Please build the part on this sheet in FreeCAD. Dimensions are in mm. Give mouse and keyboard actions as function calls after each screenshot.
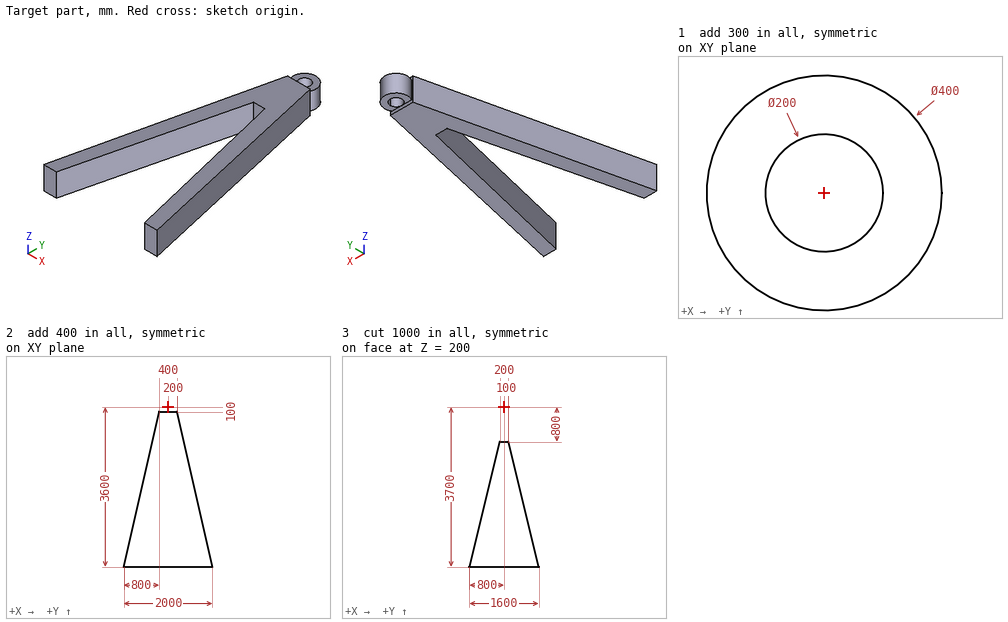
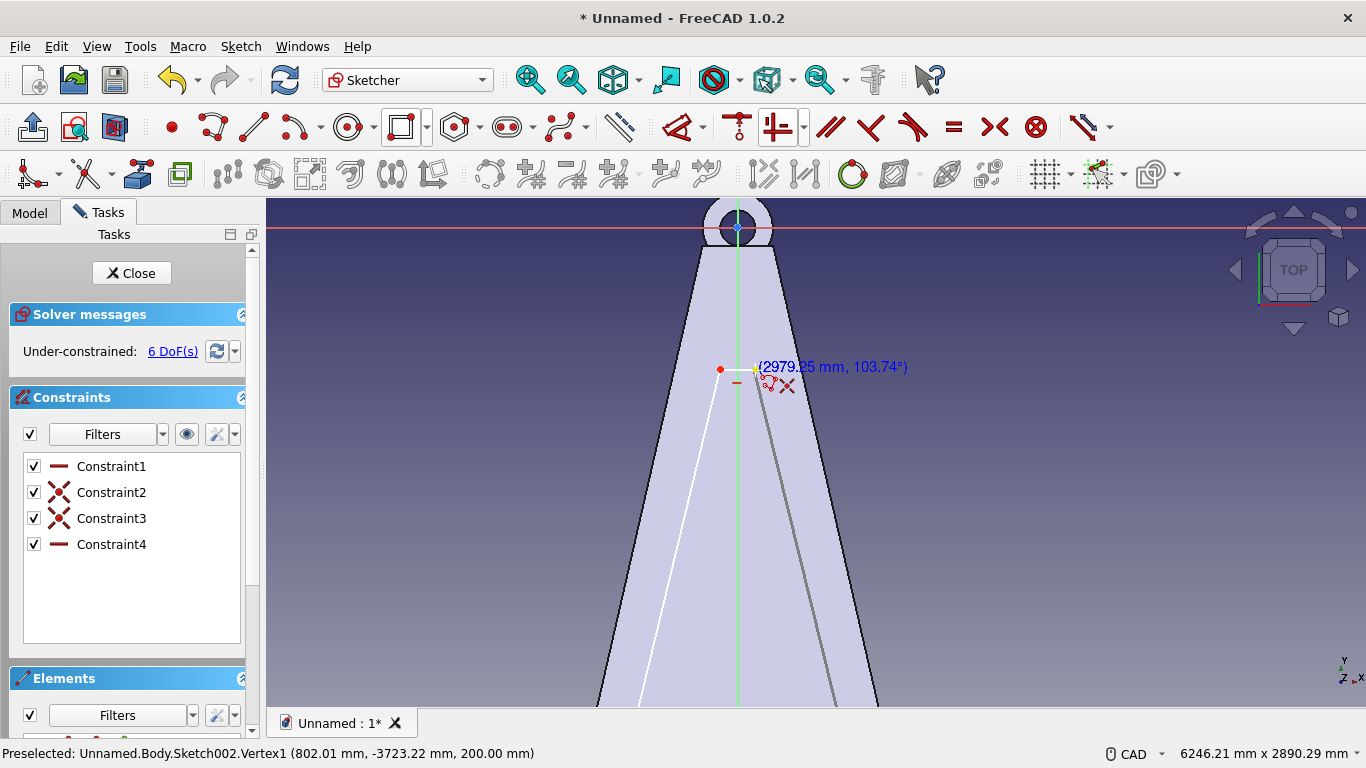
click(755, 370)
key(Escape)
key(Escape)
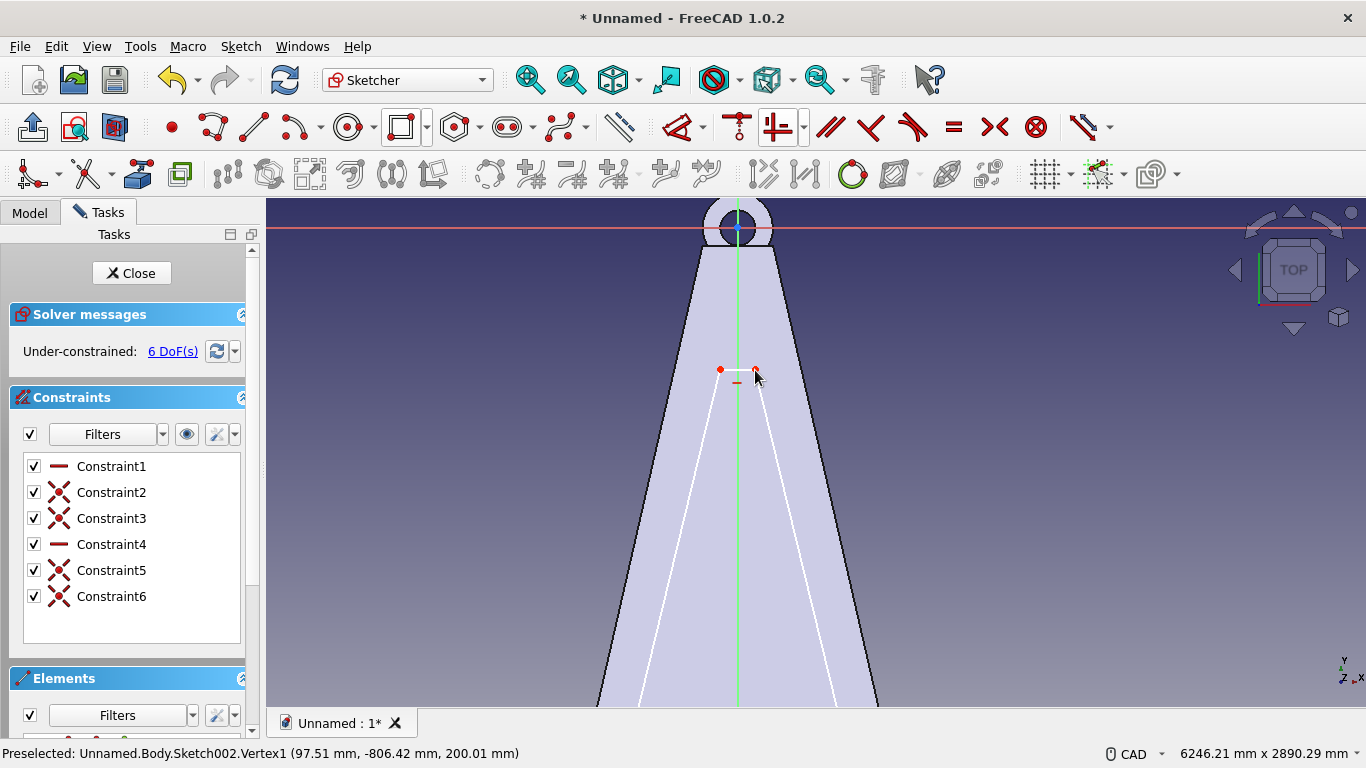
click(676, 128)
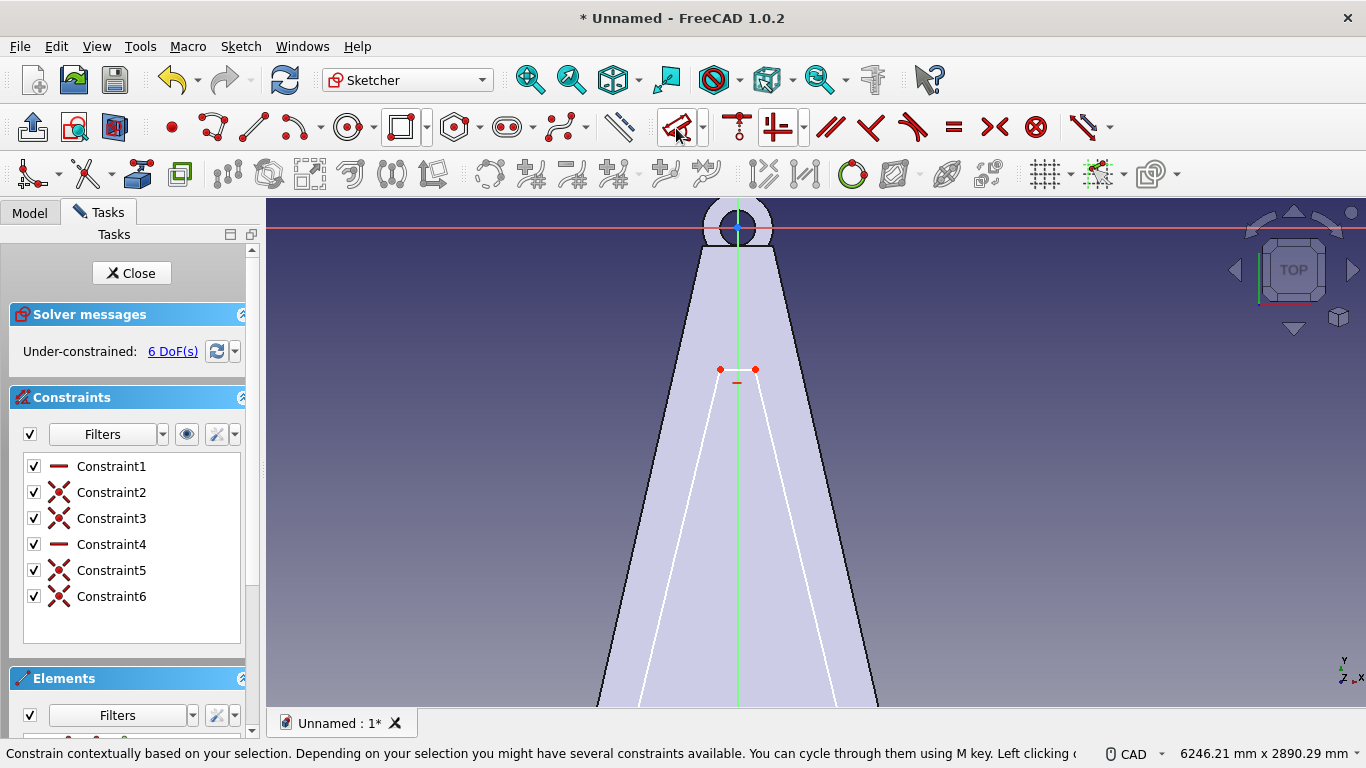
click(741, 370)
click(729, 336)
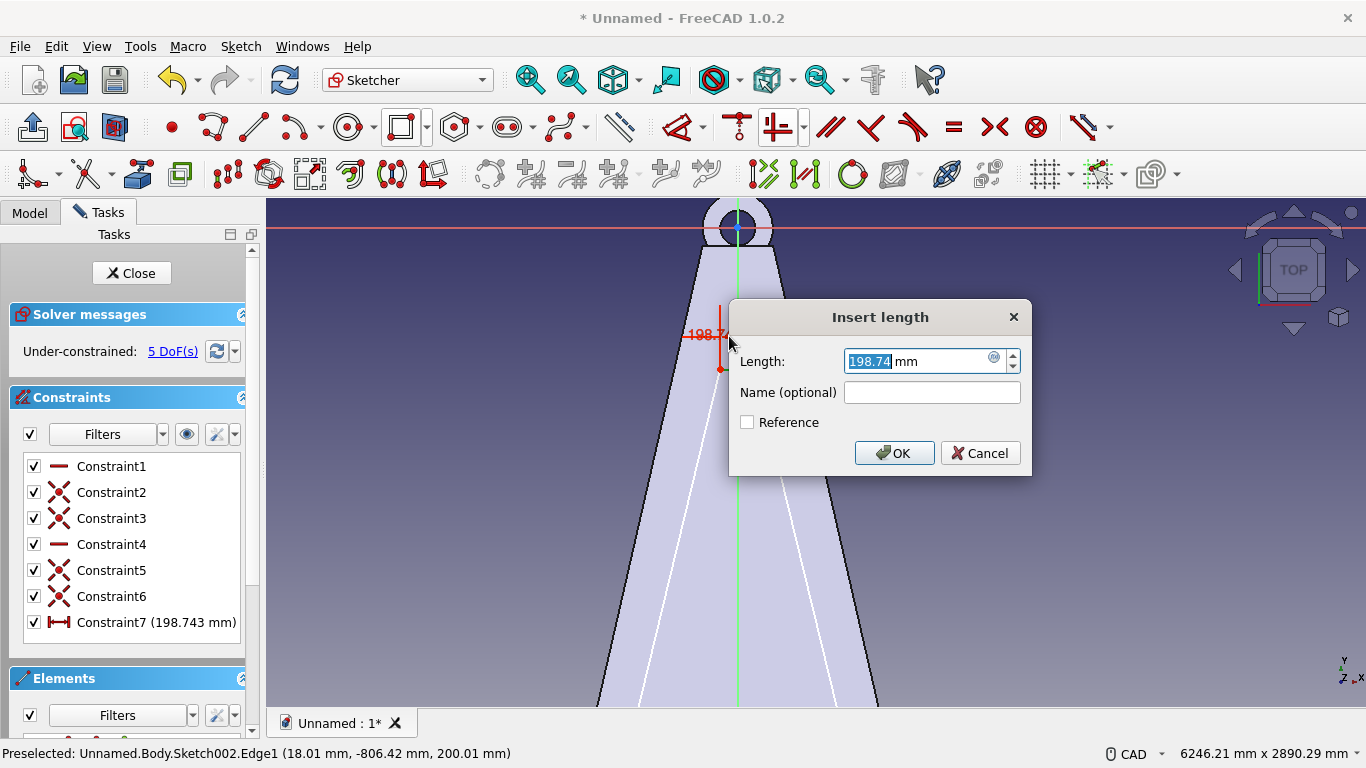
text(200)
key(Return)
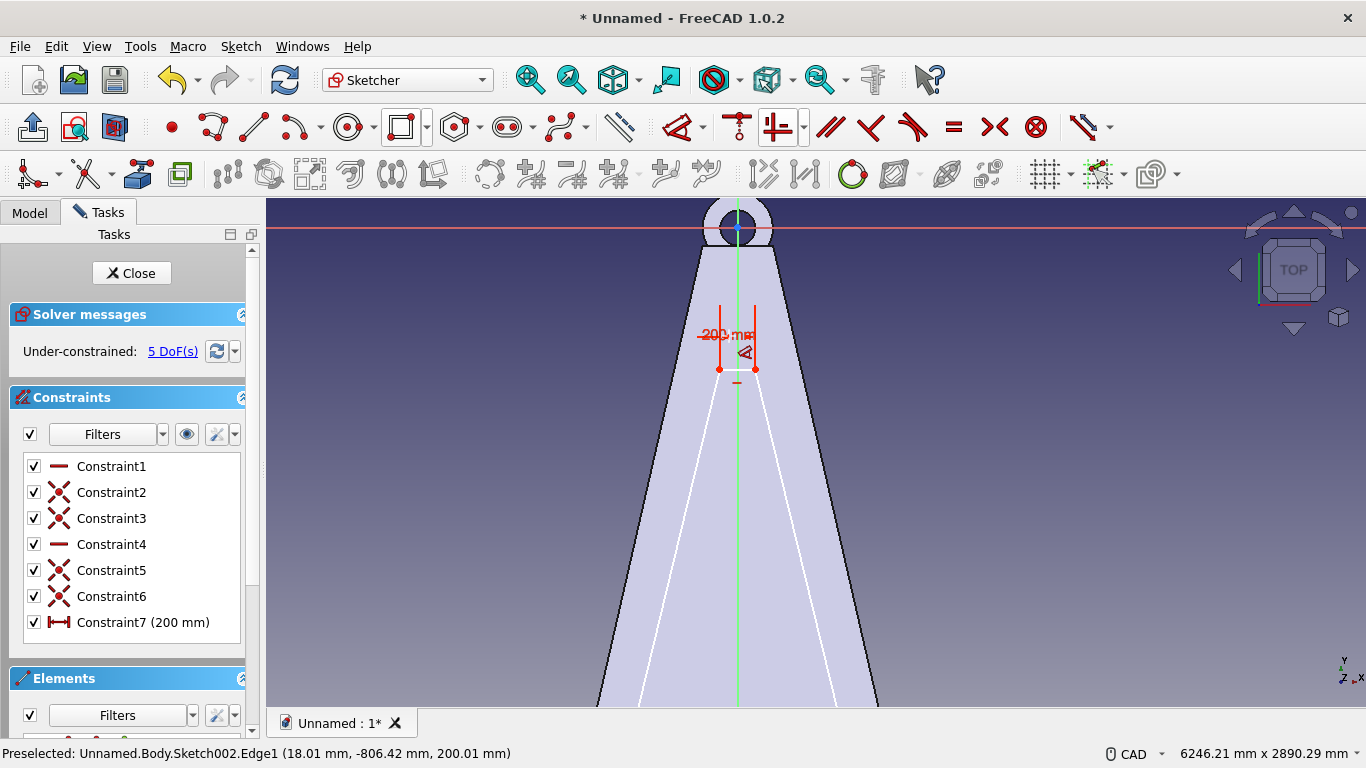
scroll(755, 370, down, 4)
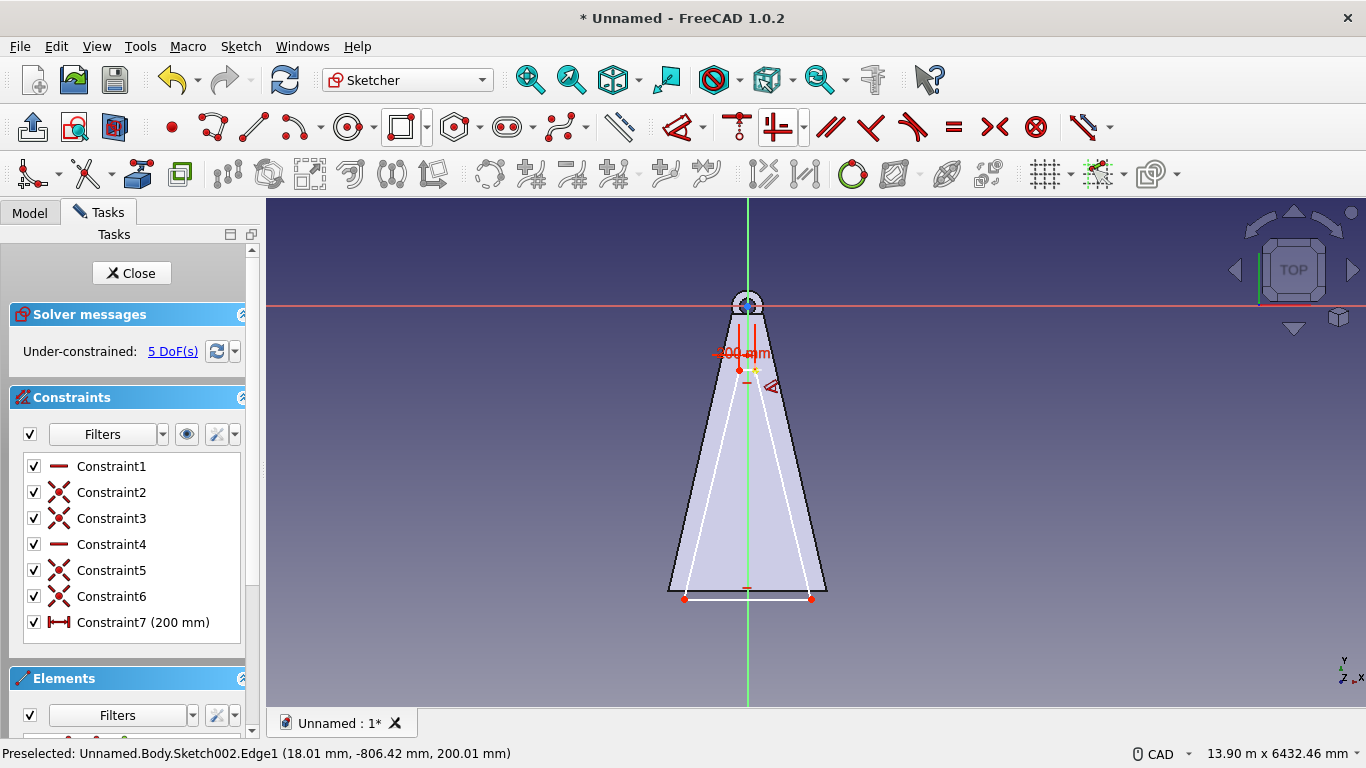
click(722, 600)
click(718, 634)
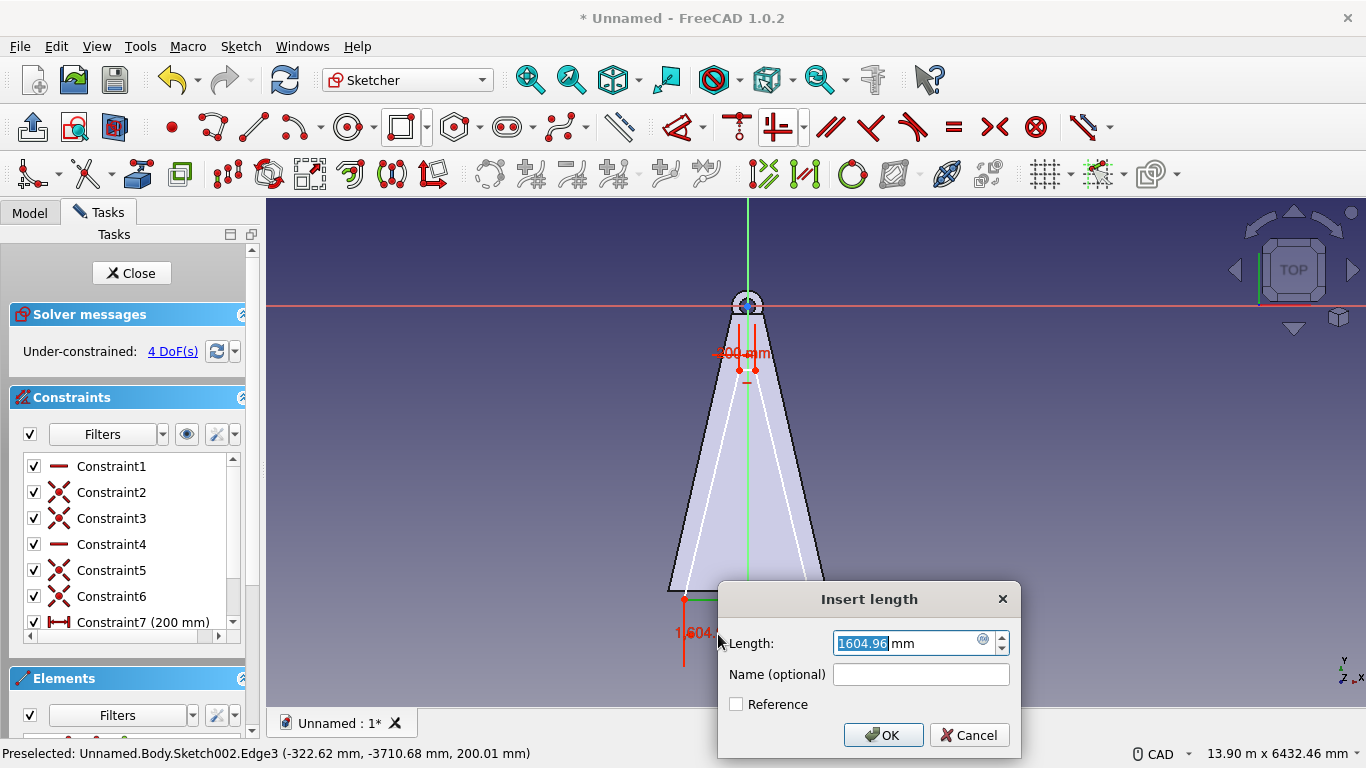
text(1600)
key(Return)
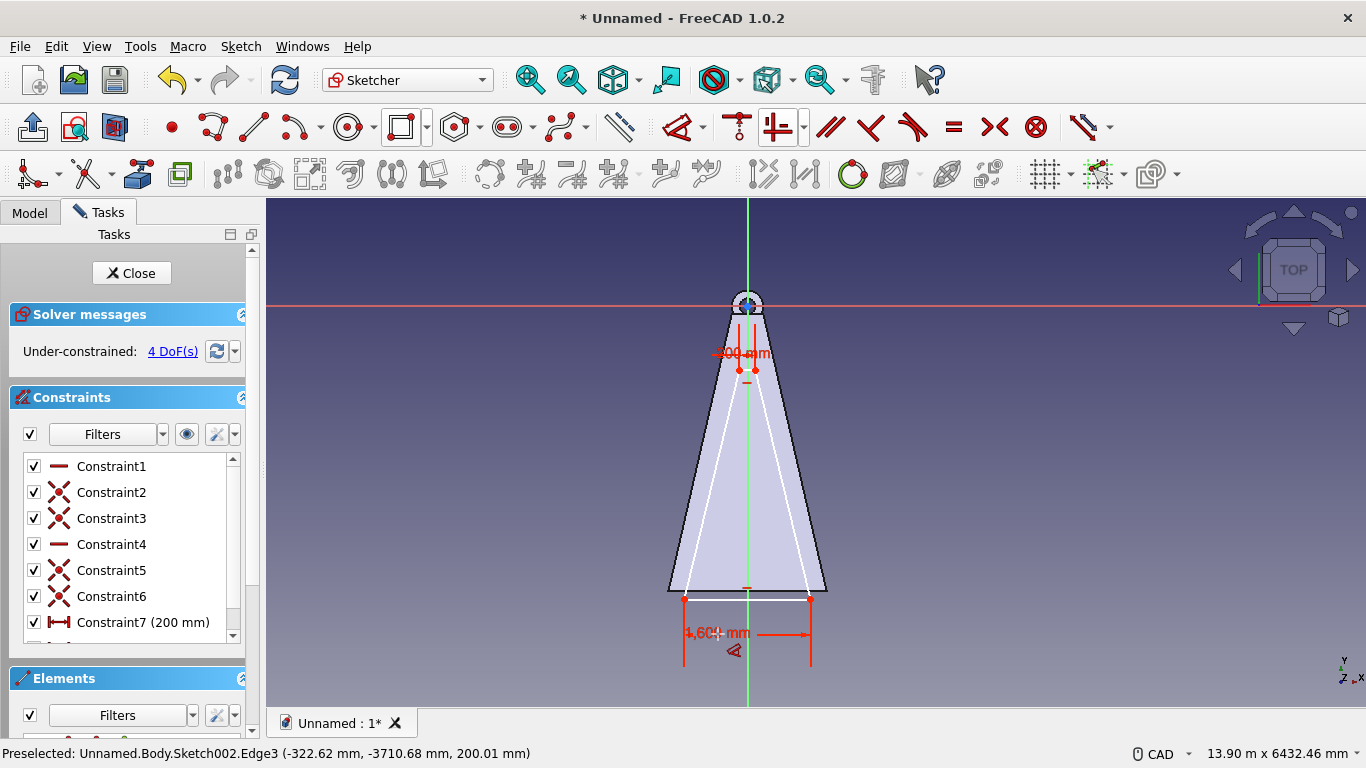
scroll(755, 370, up, 9)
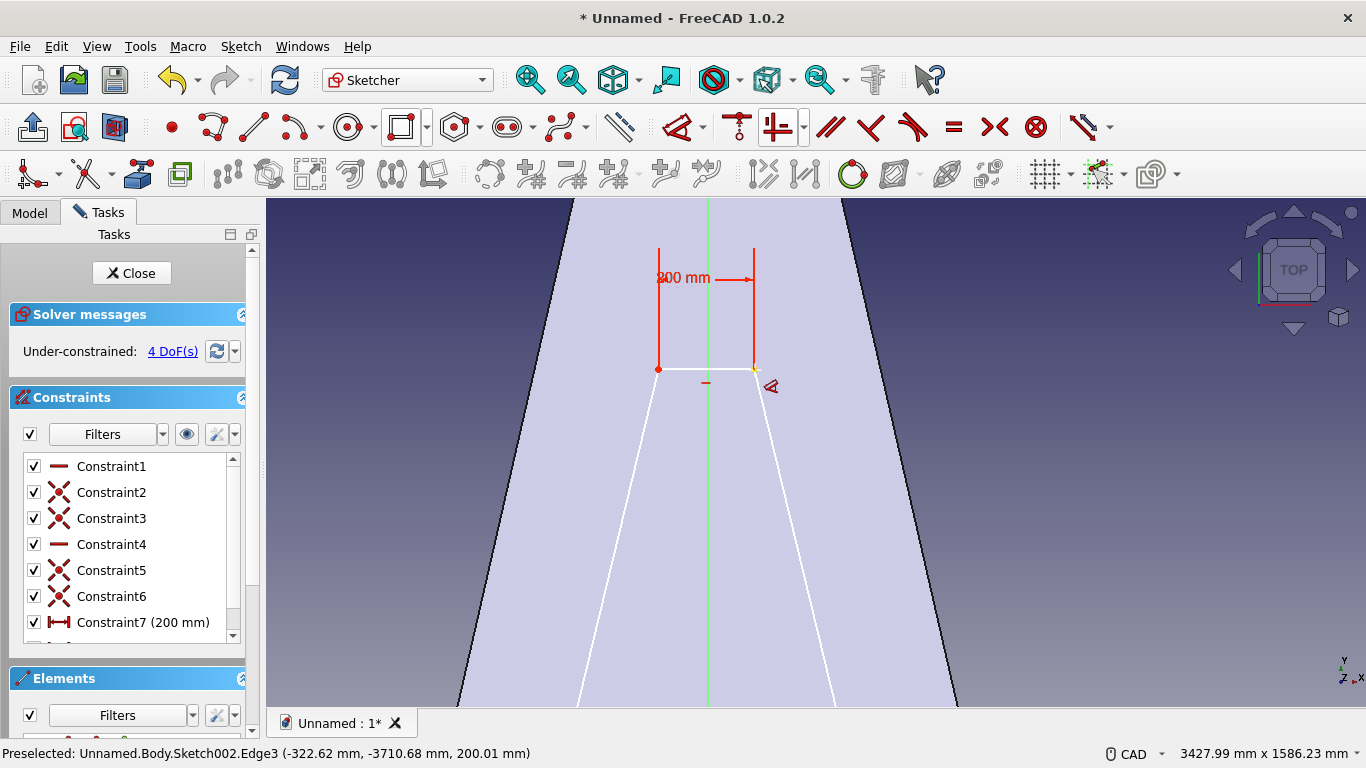
click(754, 369)
click(731, 403)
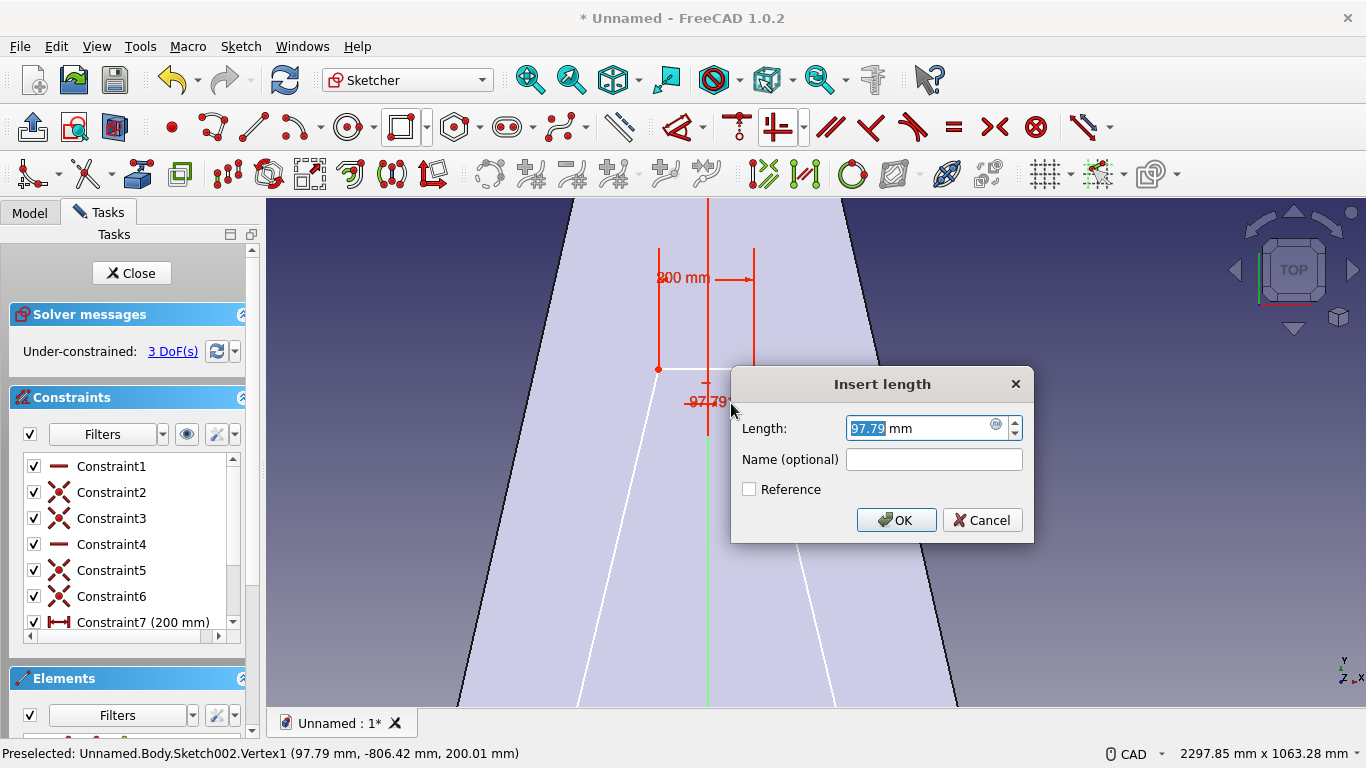
text(100)
key(Return)